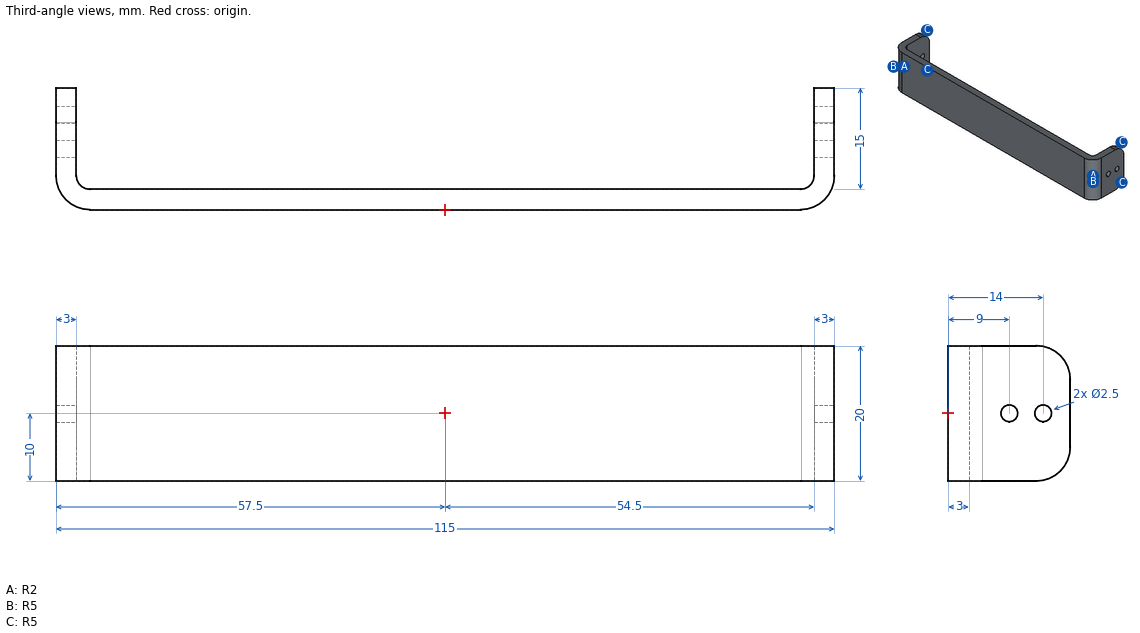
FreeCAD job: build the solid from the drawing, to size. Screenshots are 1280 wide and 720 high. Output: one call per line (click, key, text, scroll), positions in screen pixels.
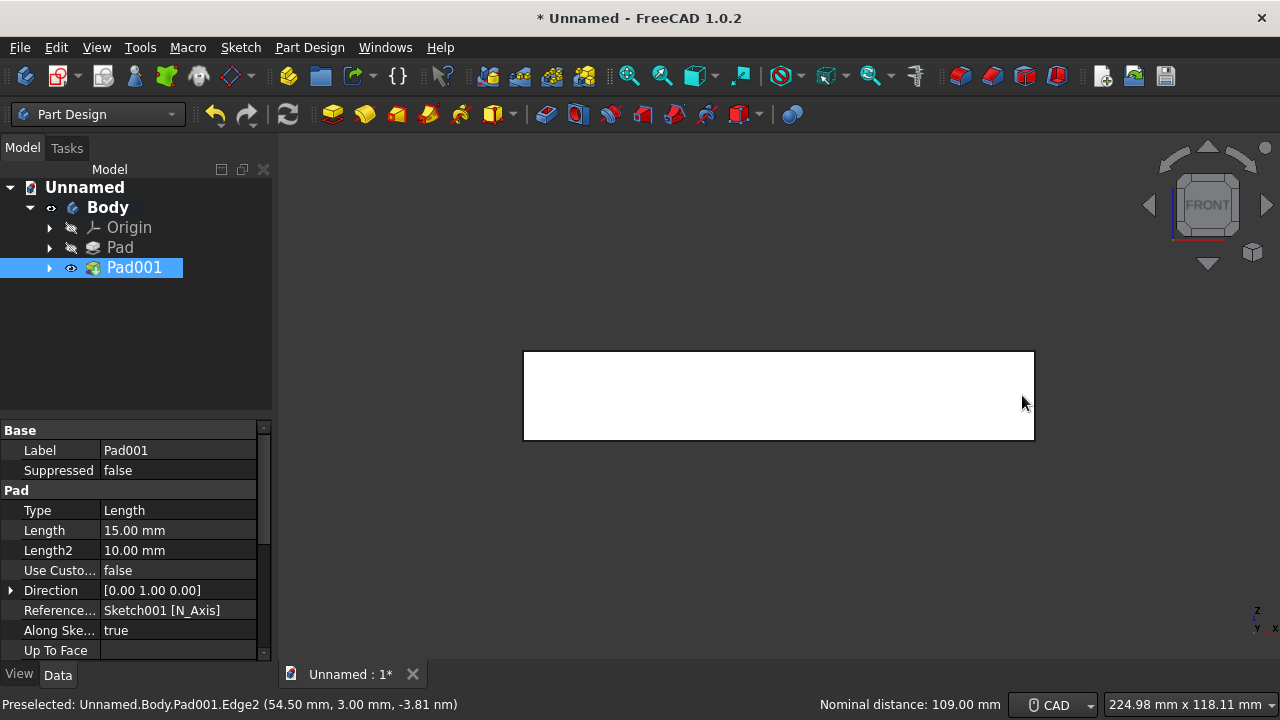
click(962, 76)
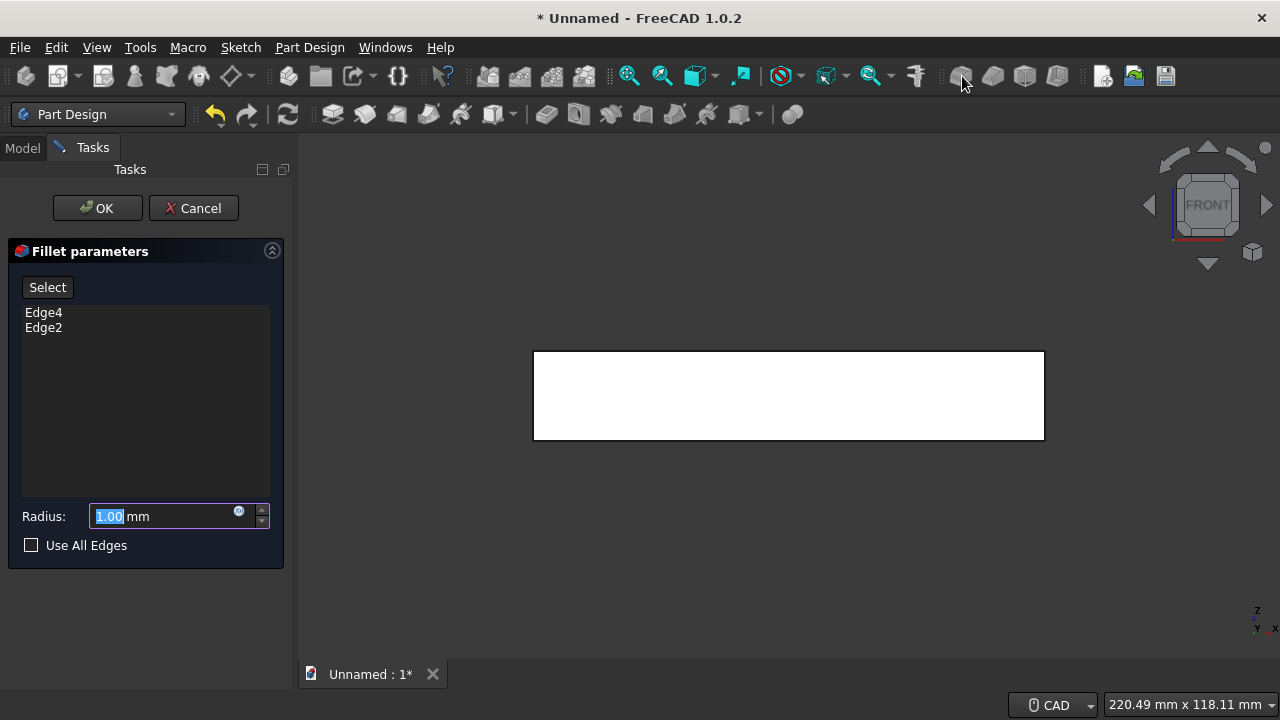
text(2)
key(Tab)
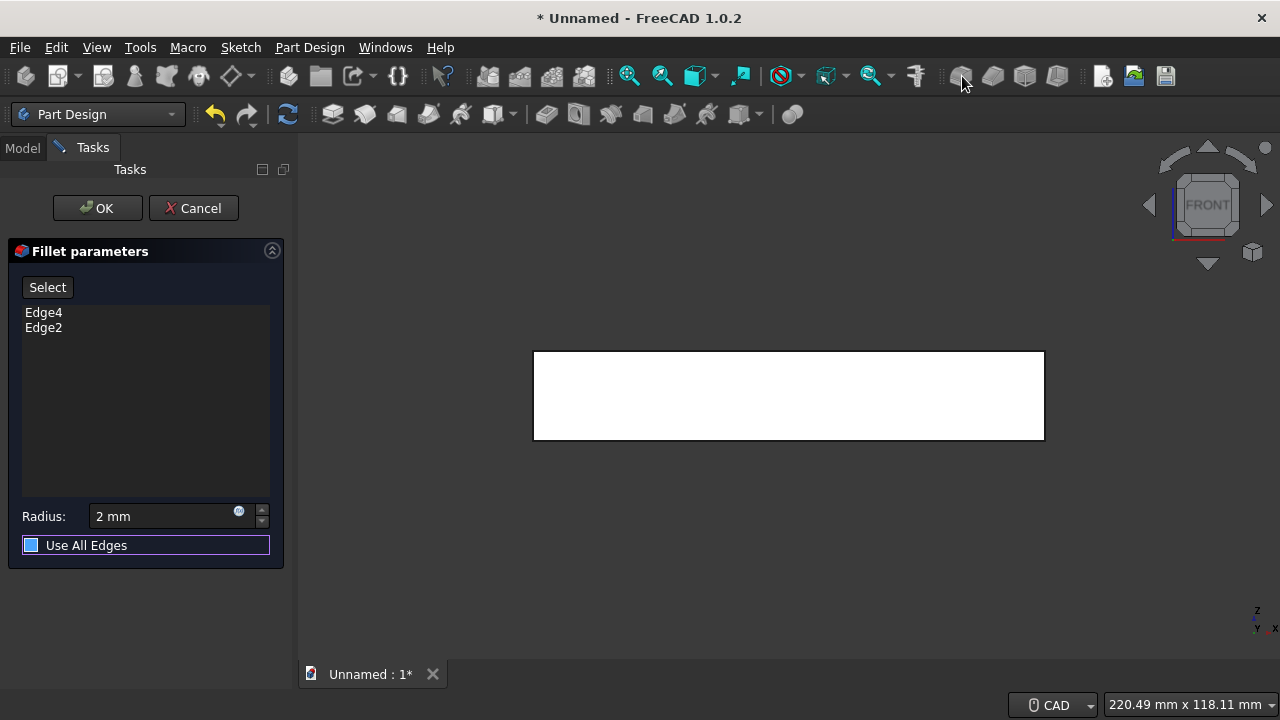
click(98, 208)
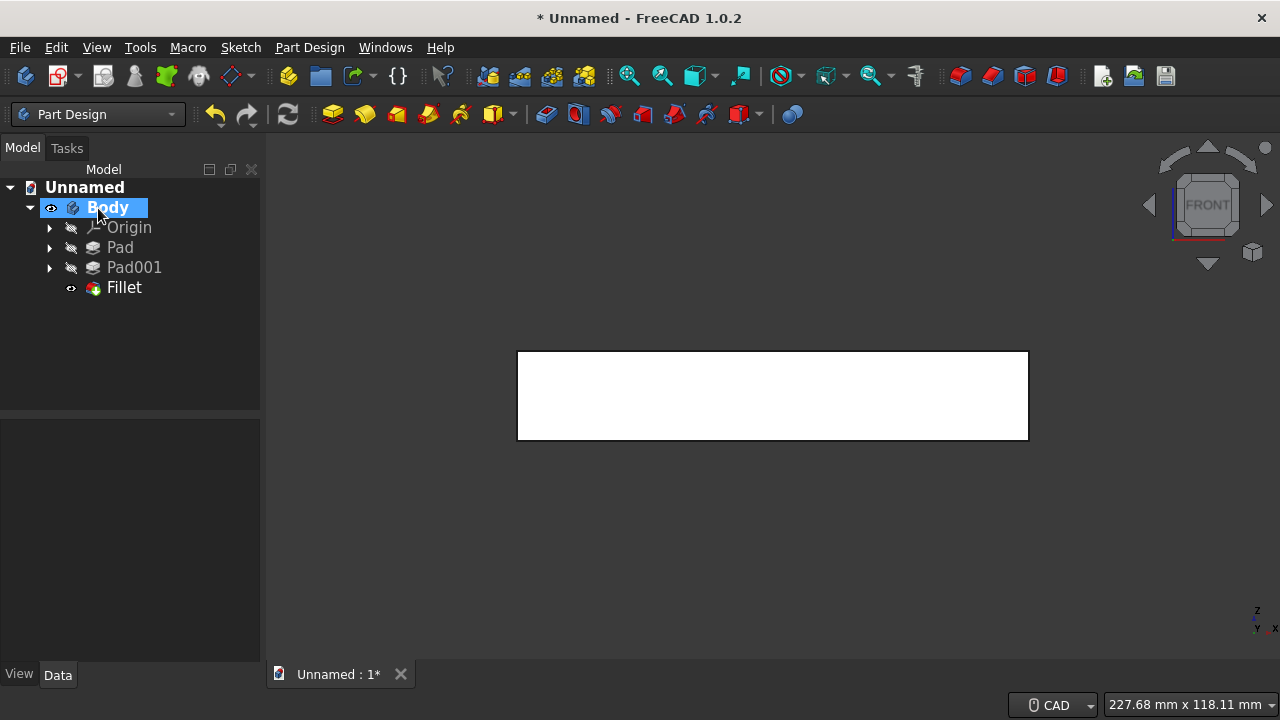
click(517, 395)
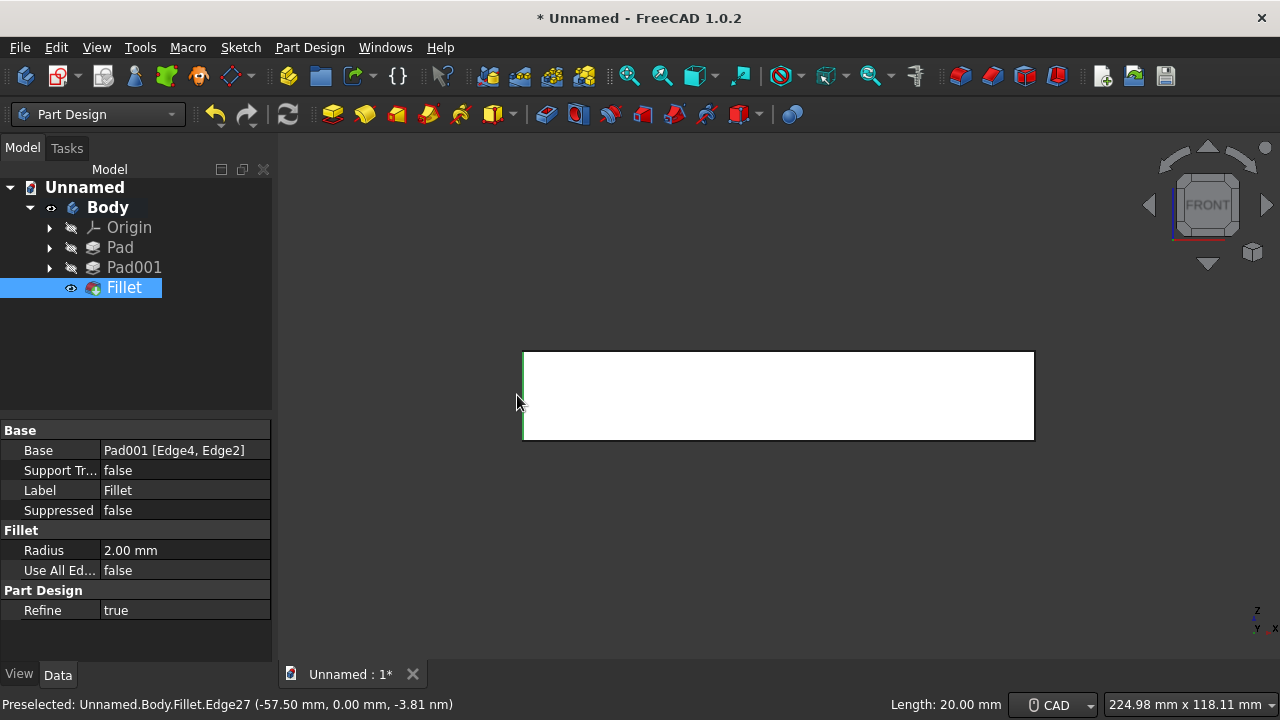
click(1035, 395, ctrl)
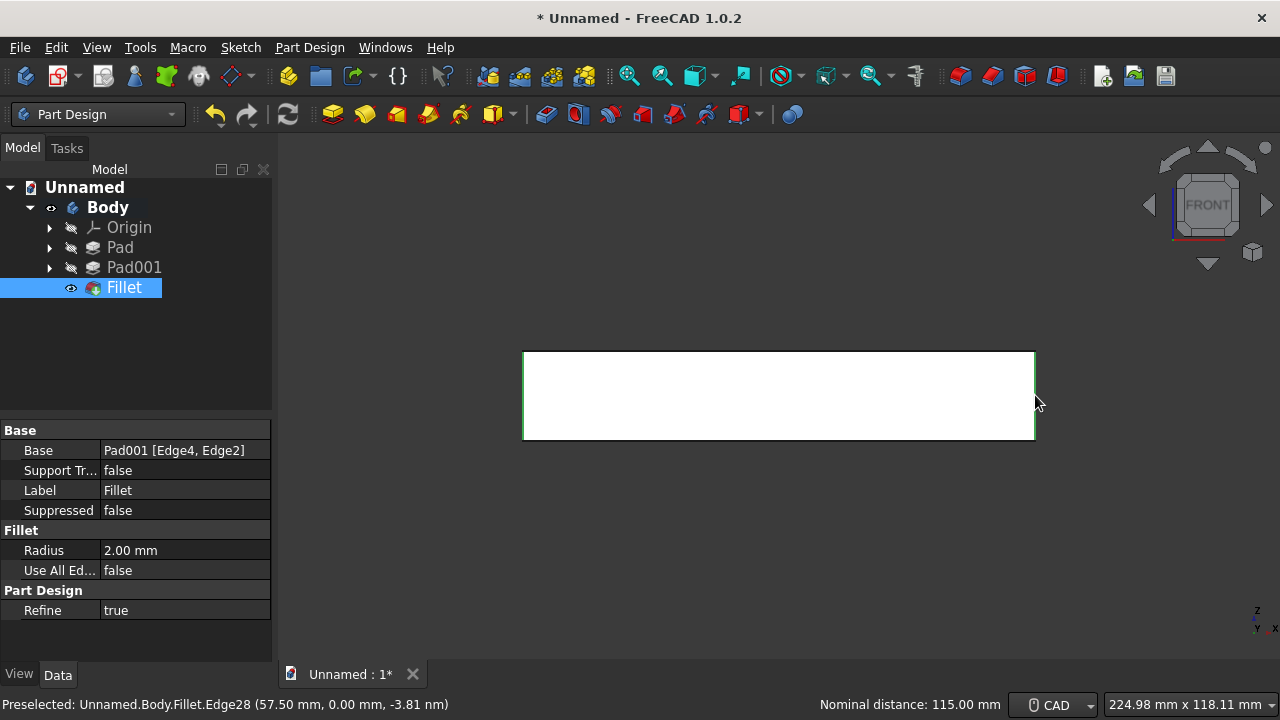
click(962, 76)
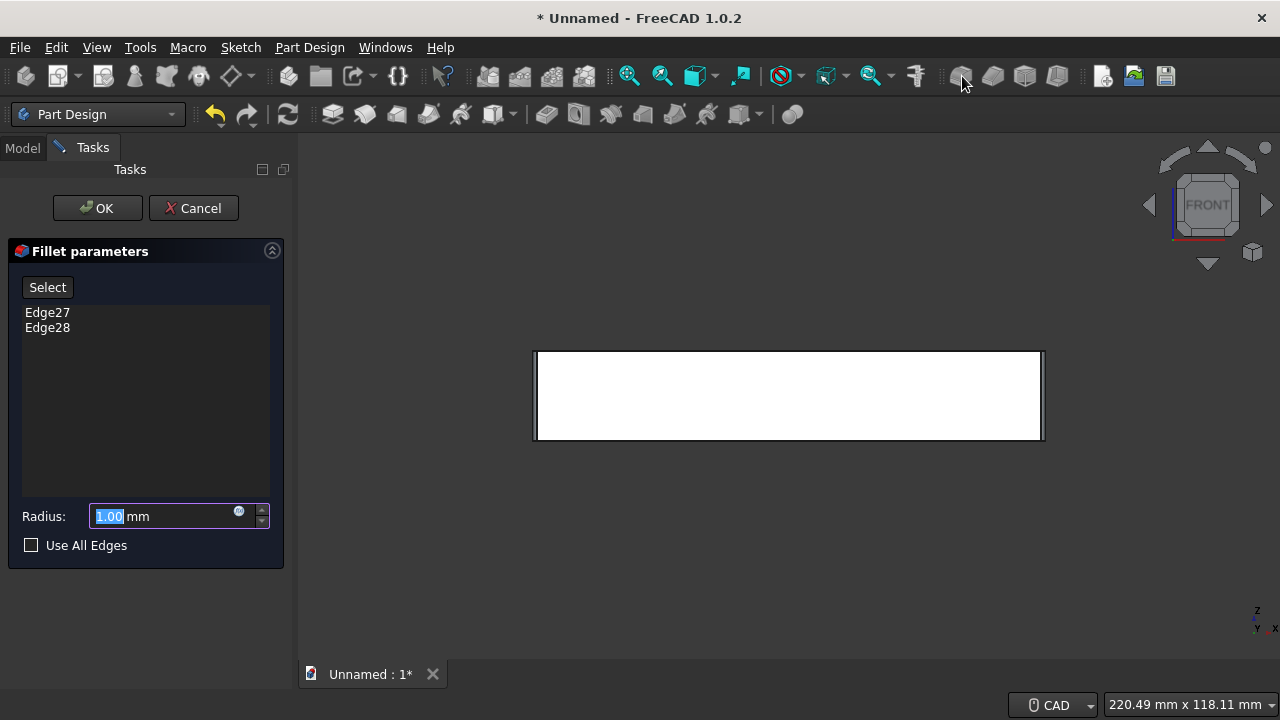
text(5)
key(Tab)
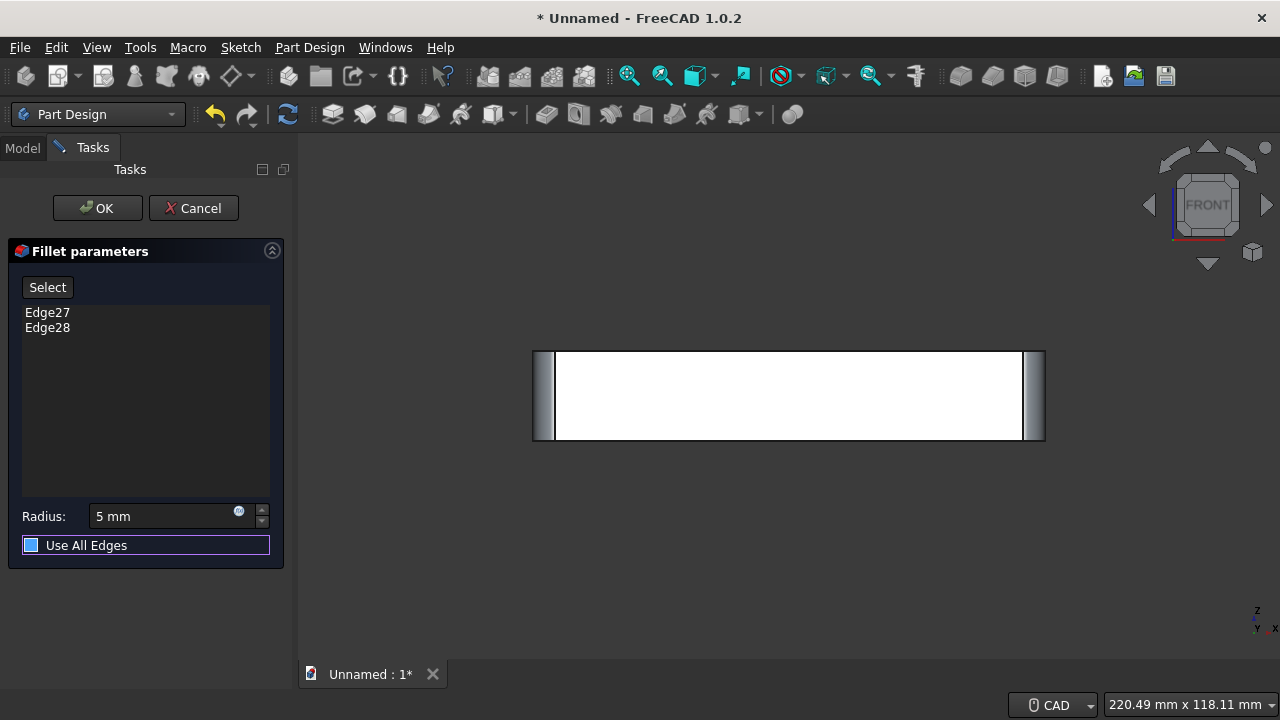
click(98, 208)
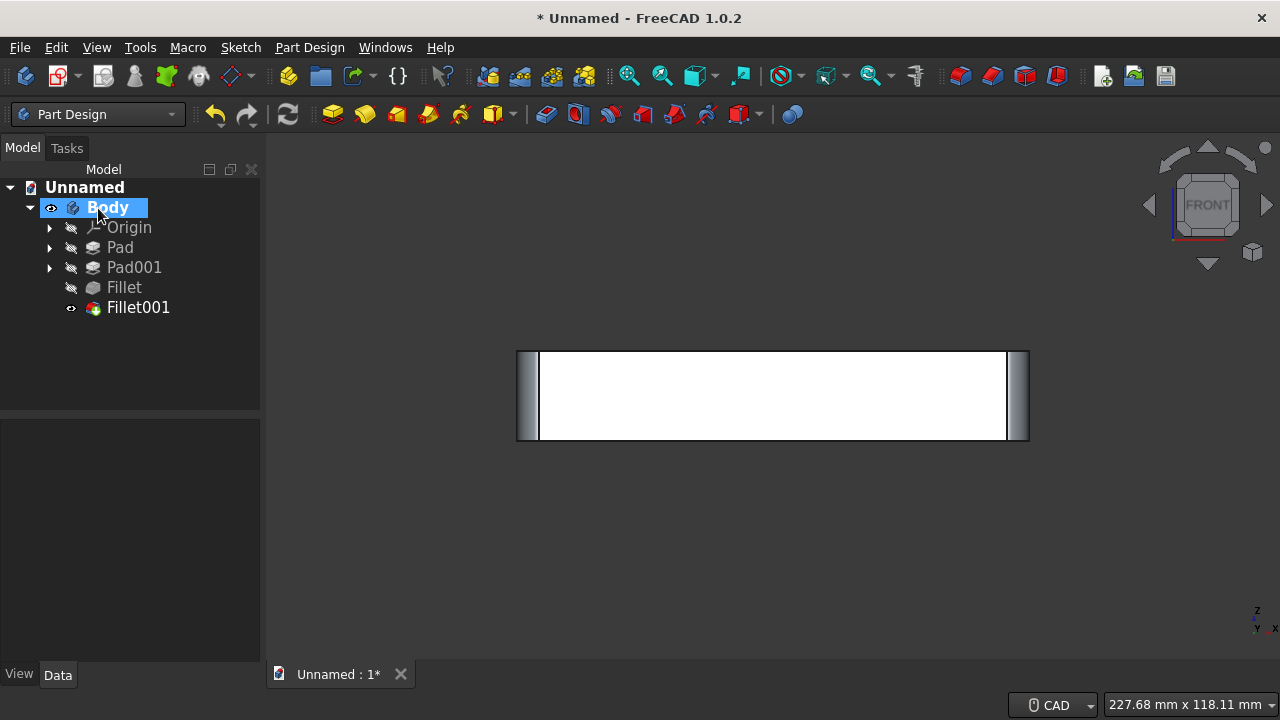
key(6)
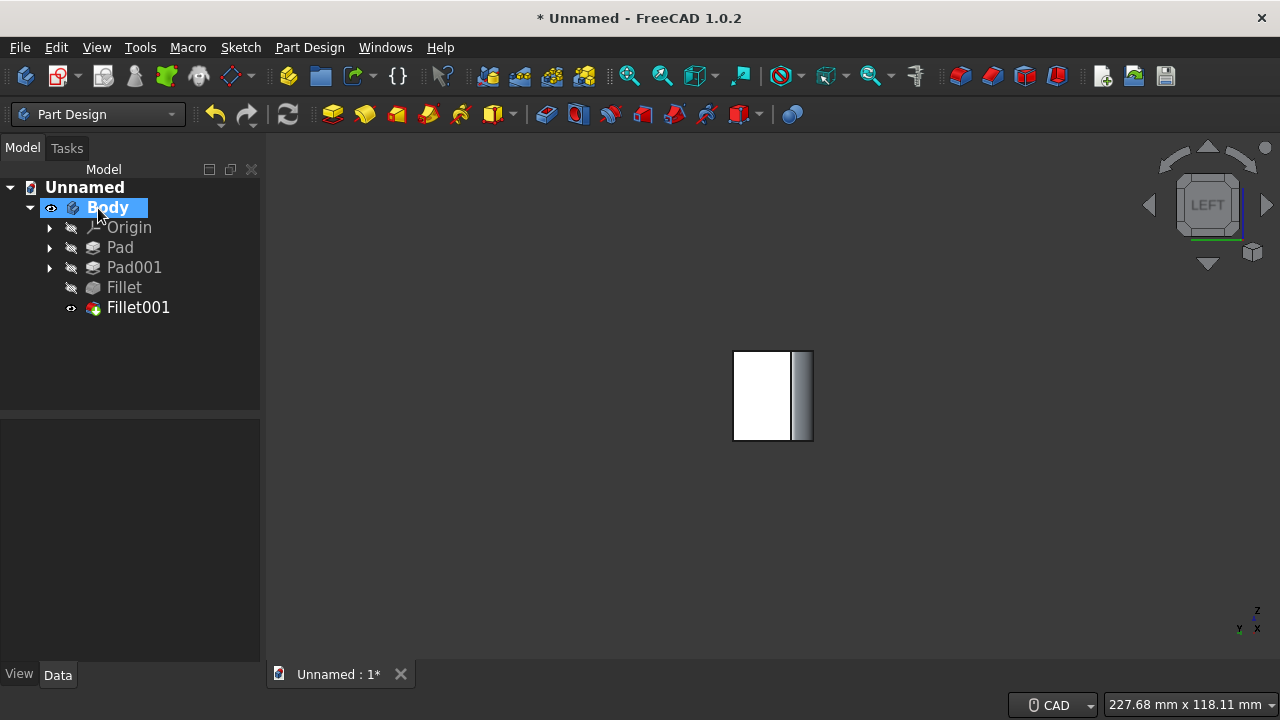
click(630, 76)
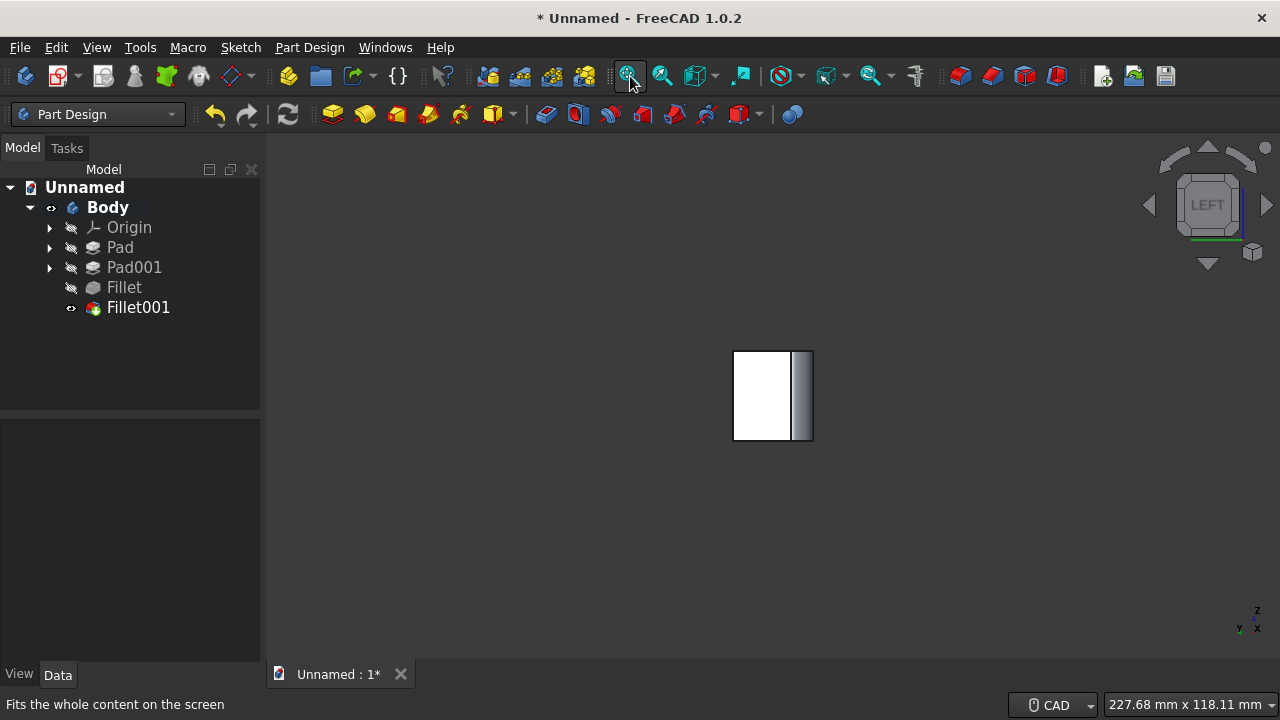
click(762, 395)